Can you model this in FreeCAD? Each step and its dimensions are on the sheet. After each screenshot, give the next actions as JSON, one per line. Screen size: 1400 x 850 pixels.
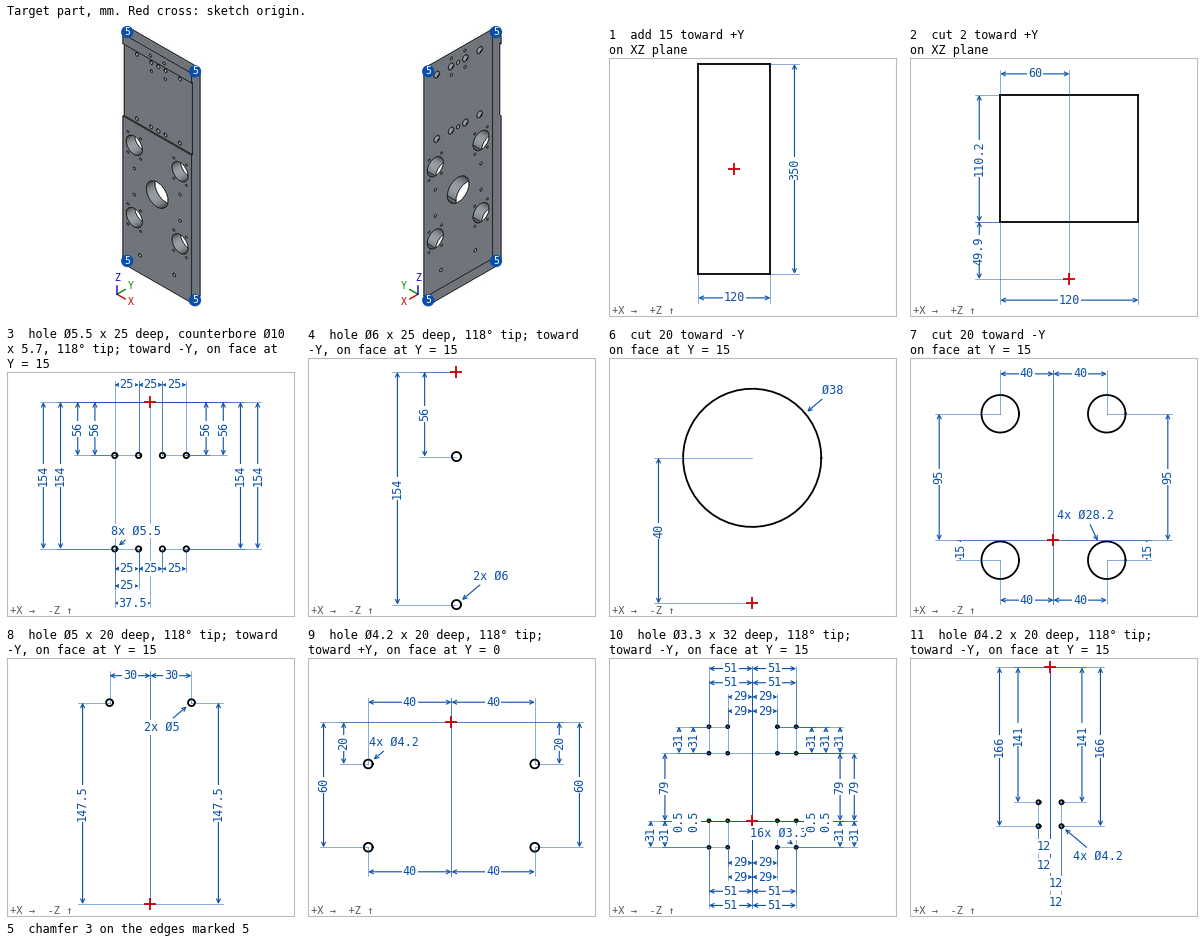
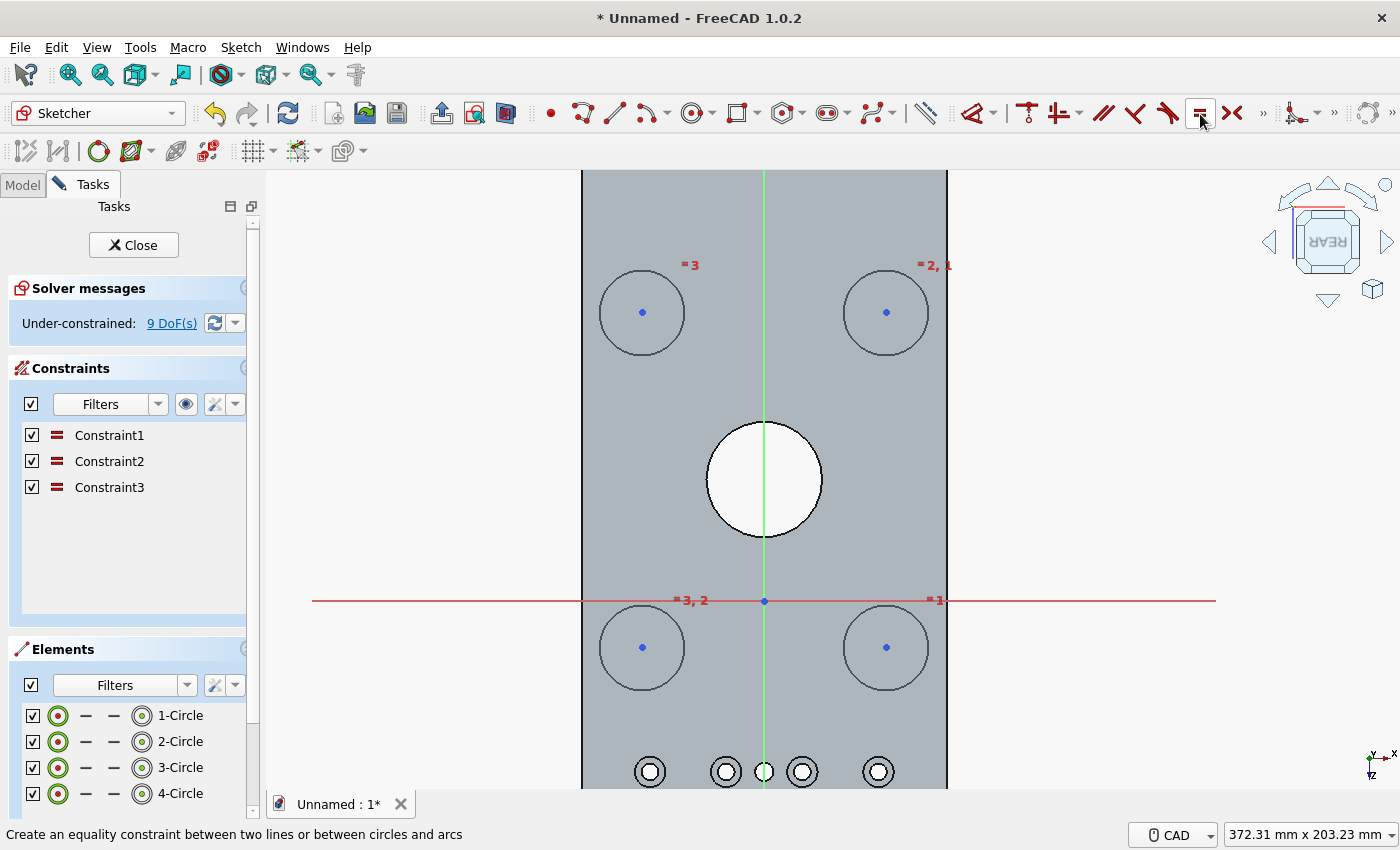
{"action": "key", "text": "d"}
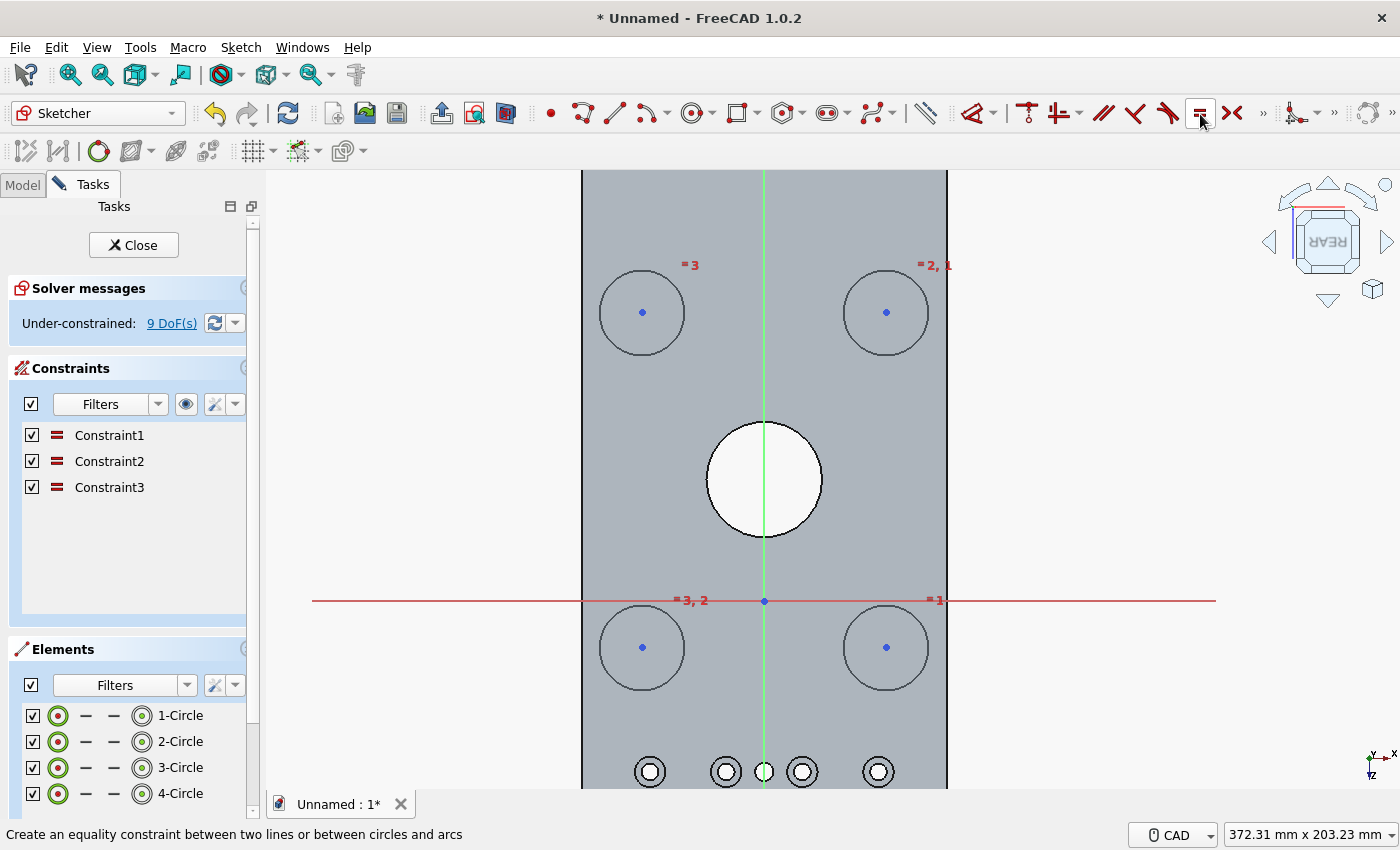
{"action": "left_click", "coordinate": [916, 618]}
{"action": "left_click", "coordinate": [957, 627]}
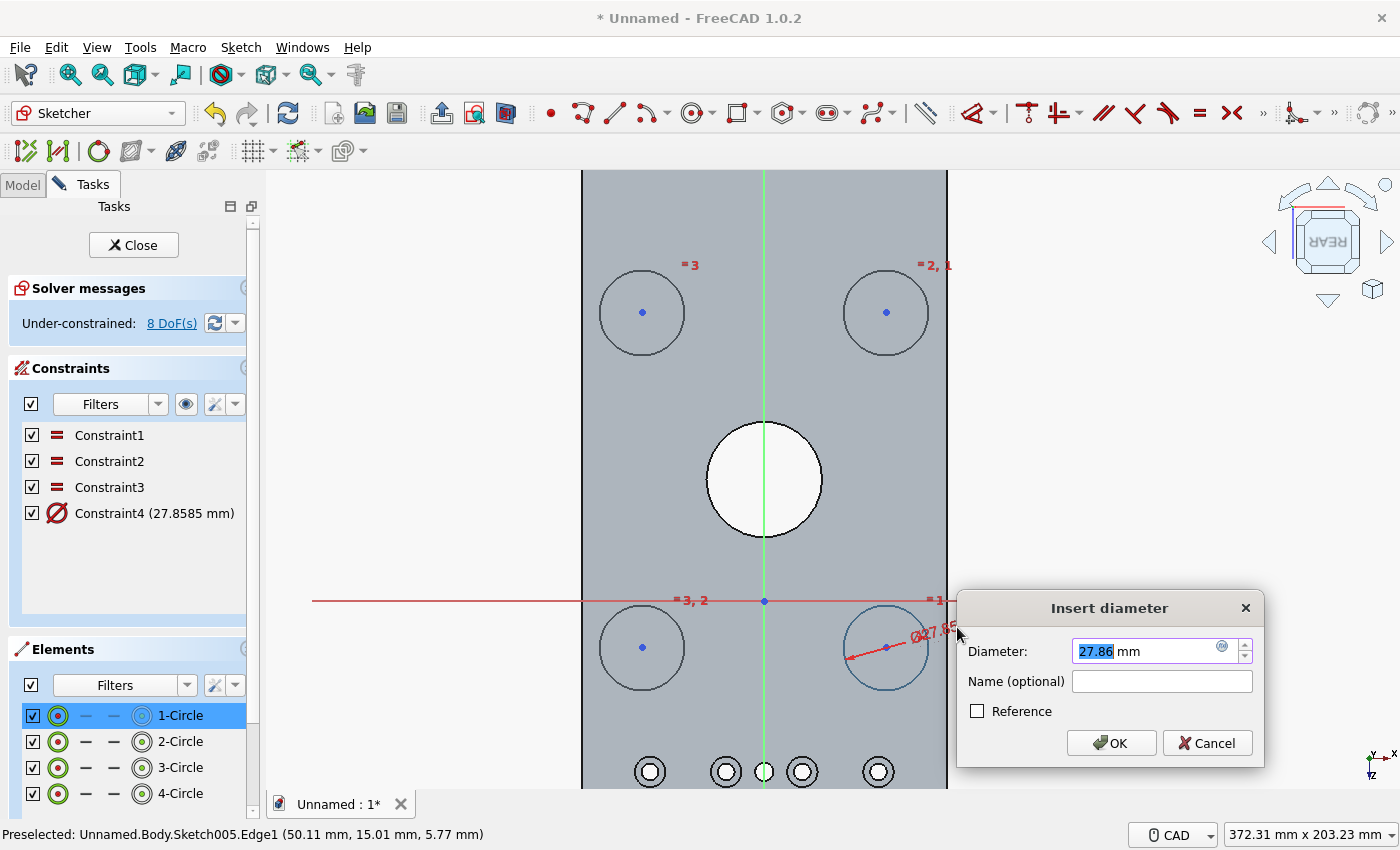
{"action": "type", "text": "28.2"}
{"action": "key", "text": "Return"}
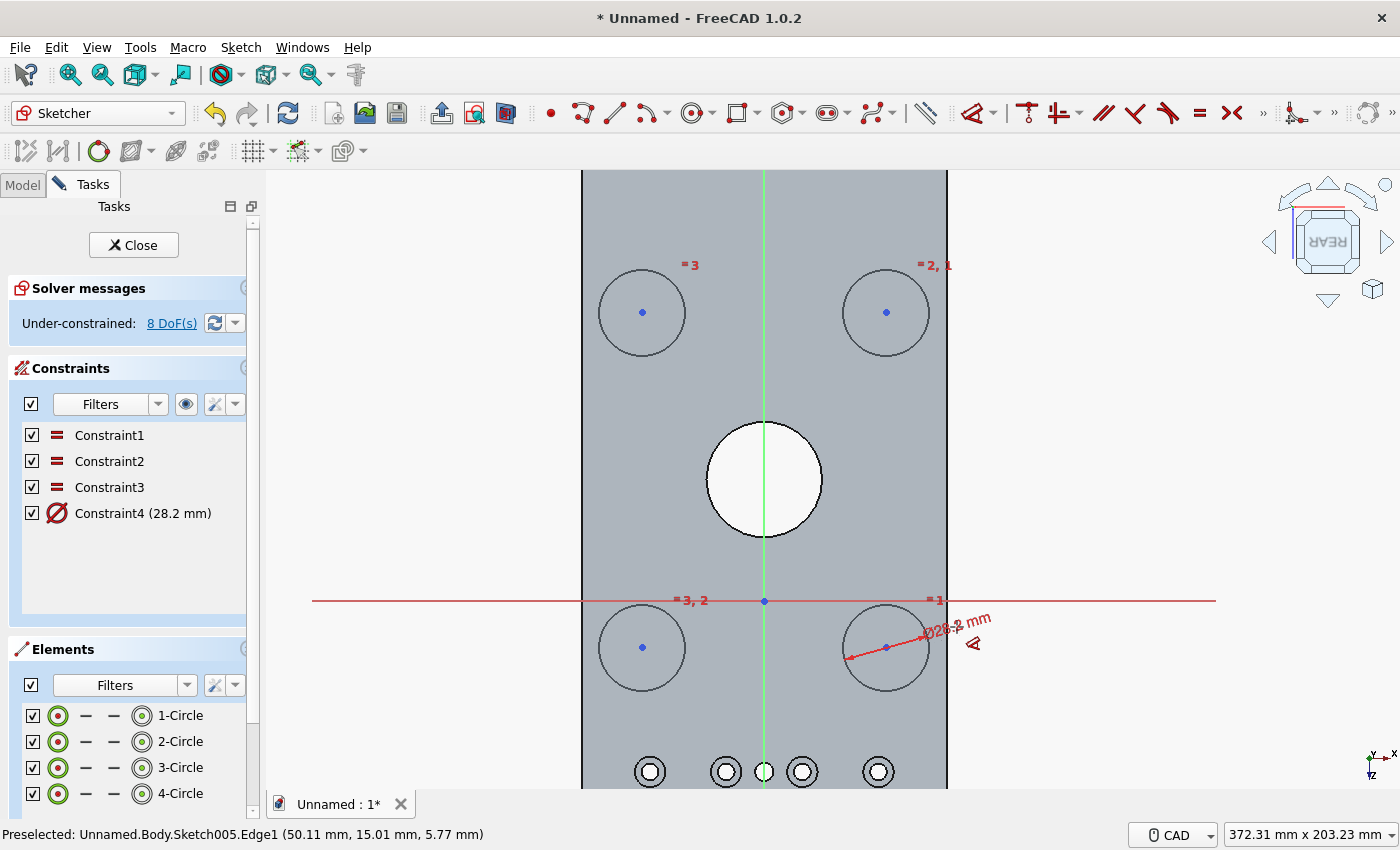
{"action": "left_click", "coordinate": [886, 648]}
{"action": "left_click", "coordinate": [825, 682]}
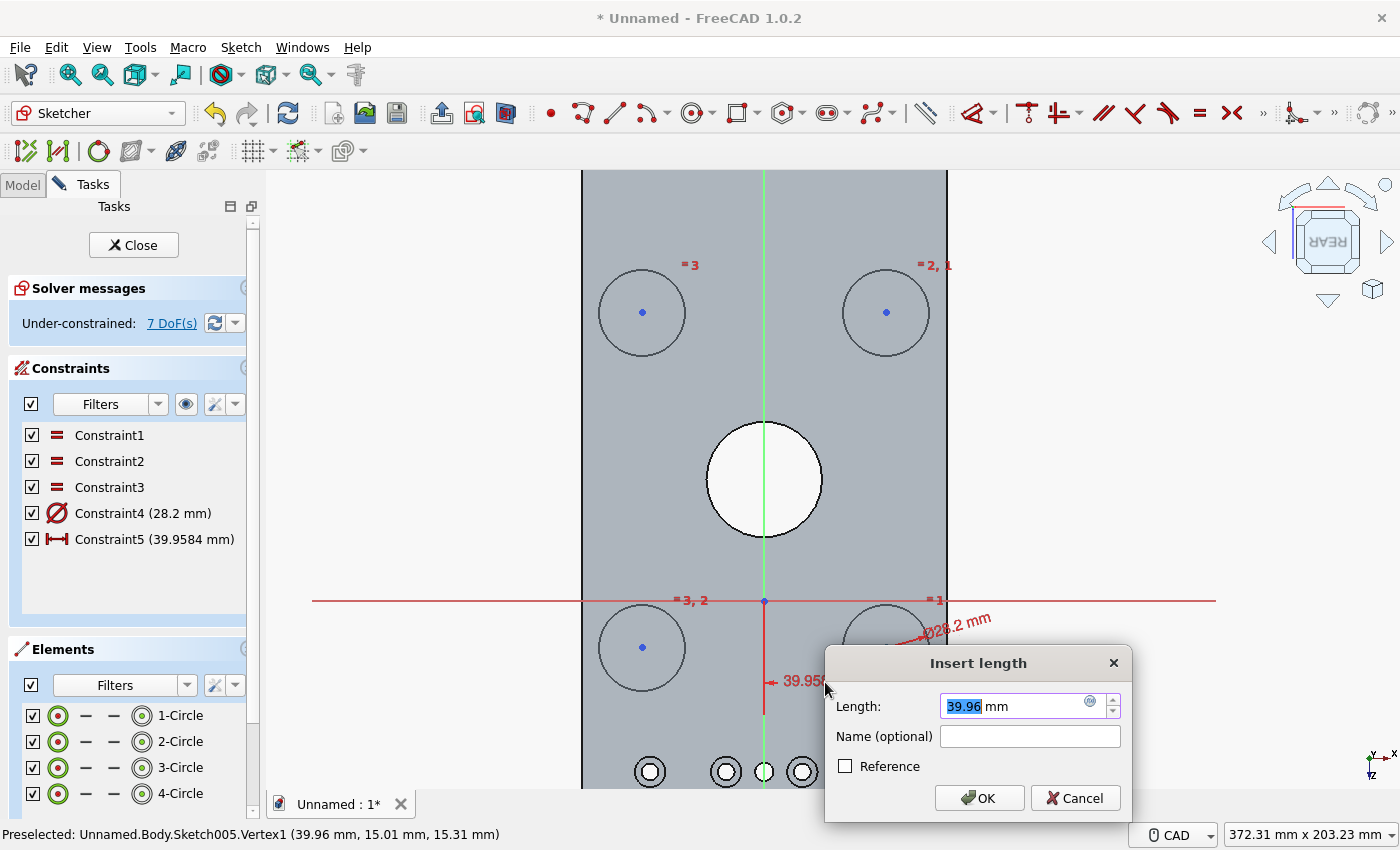
{"action": "type", "text": "40"}
{"action": "key", "text": "Return"}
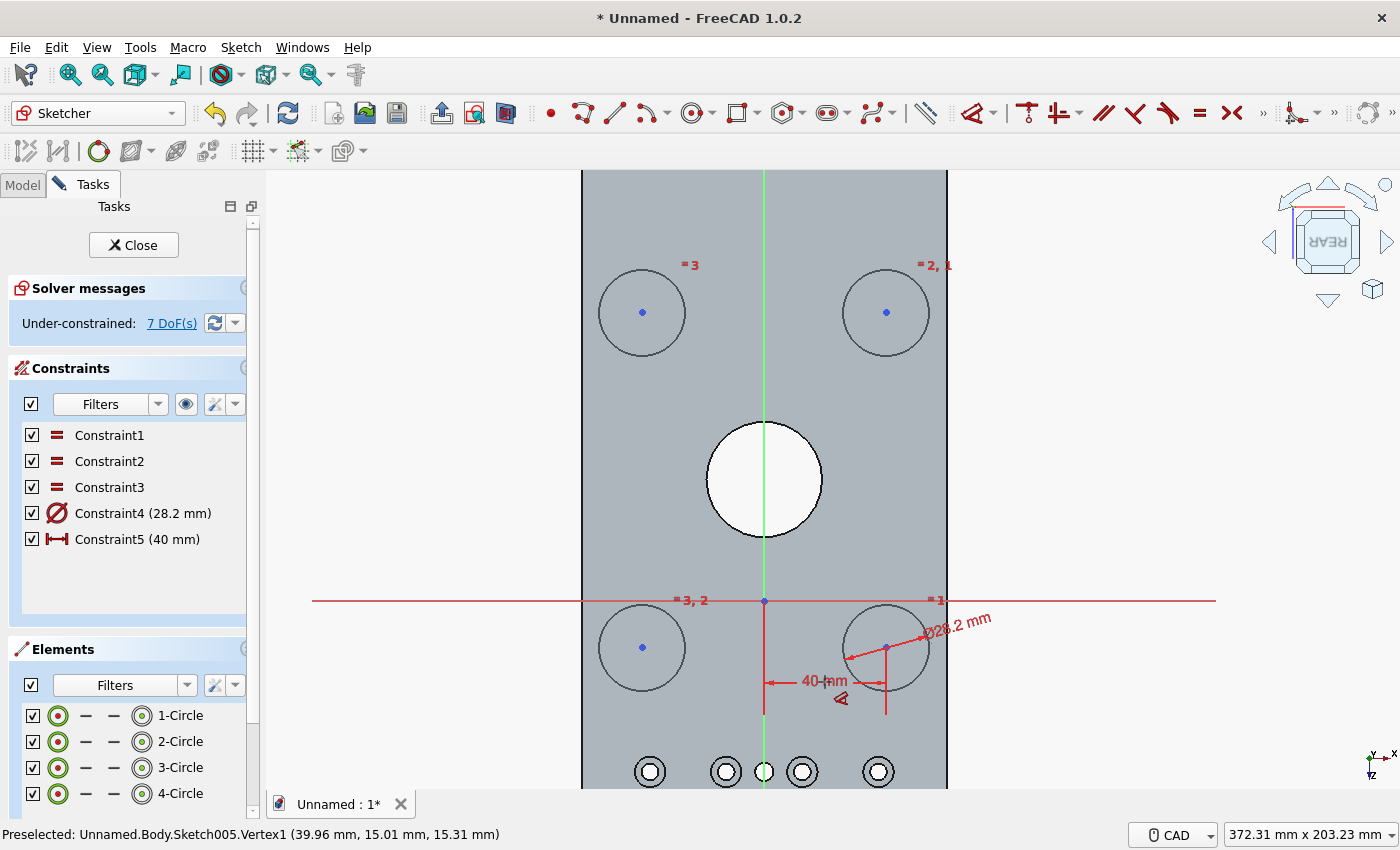
{"action": "left_click", "coordinate": [886, 648]}
{"action": "left_click", "coordinate": [730, 625]}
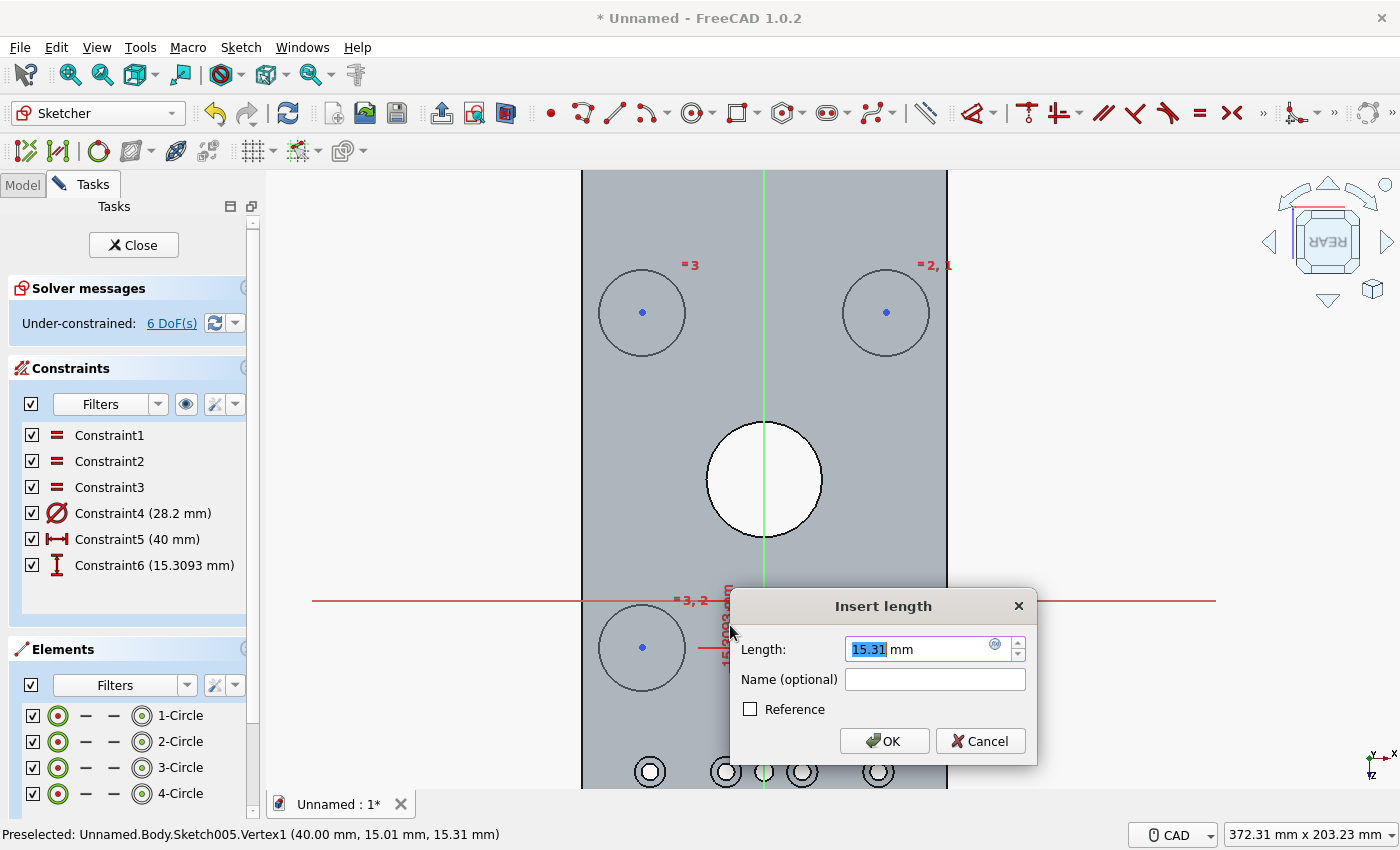
{"action": "type", "text": "15"}
{"action": "key", "text": "Return"}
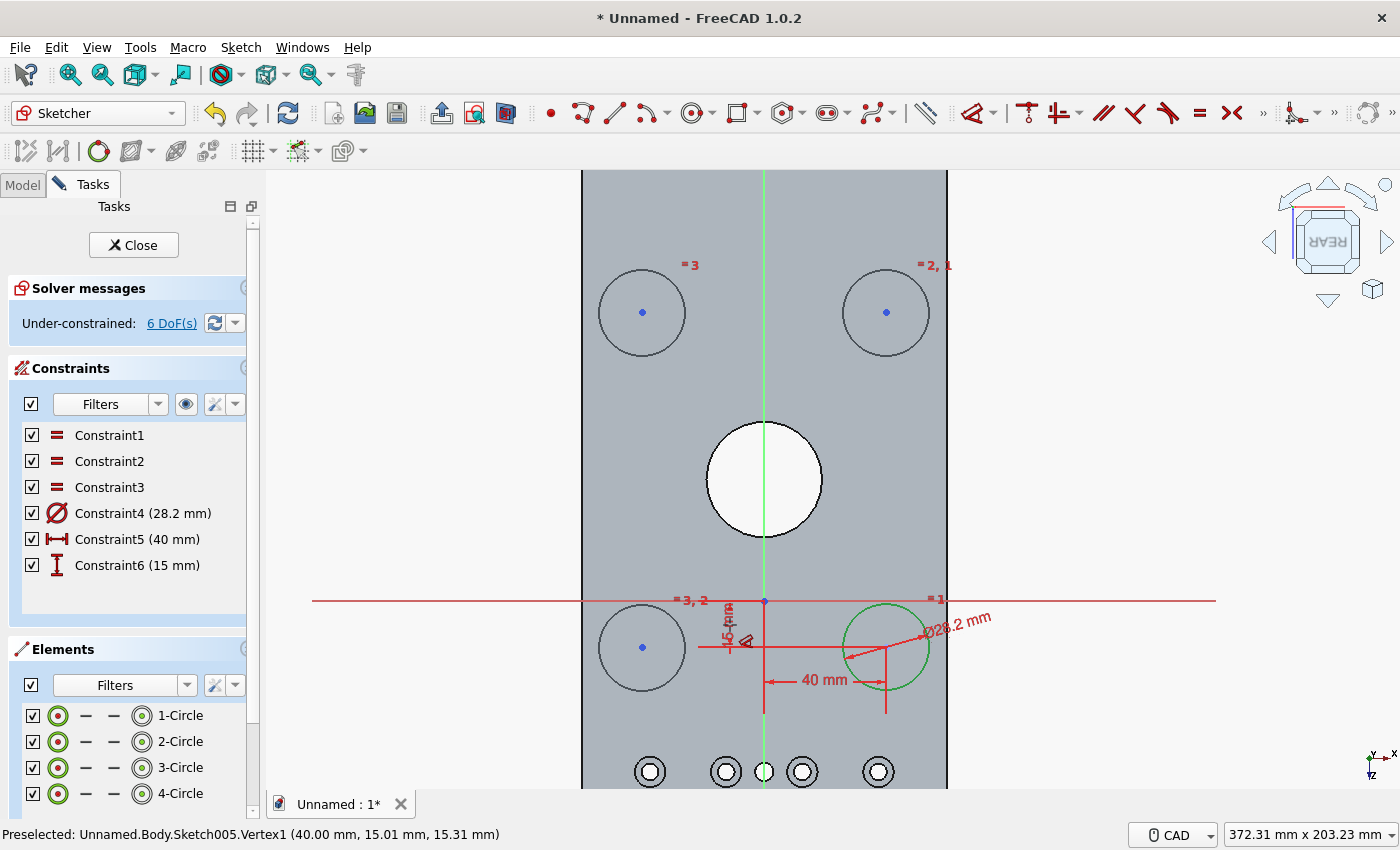
{"action": "left_click", "coordinate": [886, 313]}
{"action": "left_click", "coordinate": [825, 279]}